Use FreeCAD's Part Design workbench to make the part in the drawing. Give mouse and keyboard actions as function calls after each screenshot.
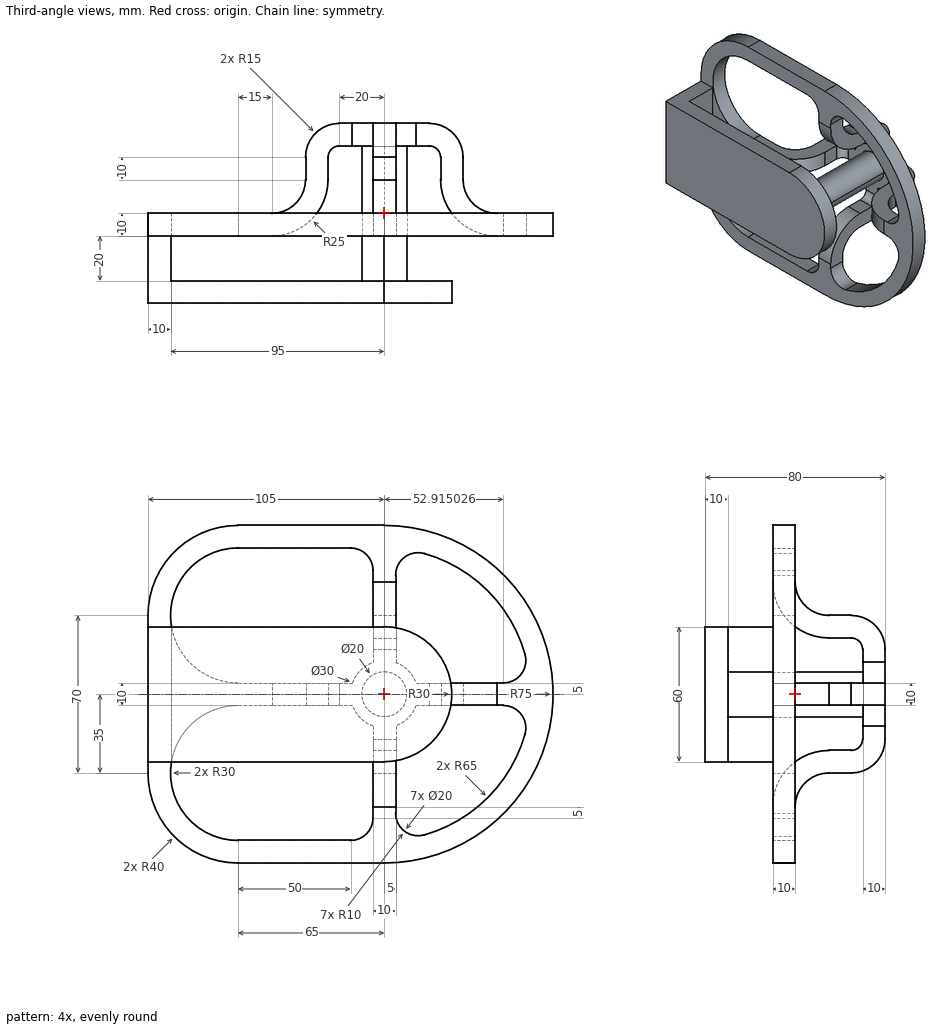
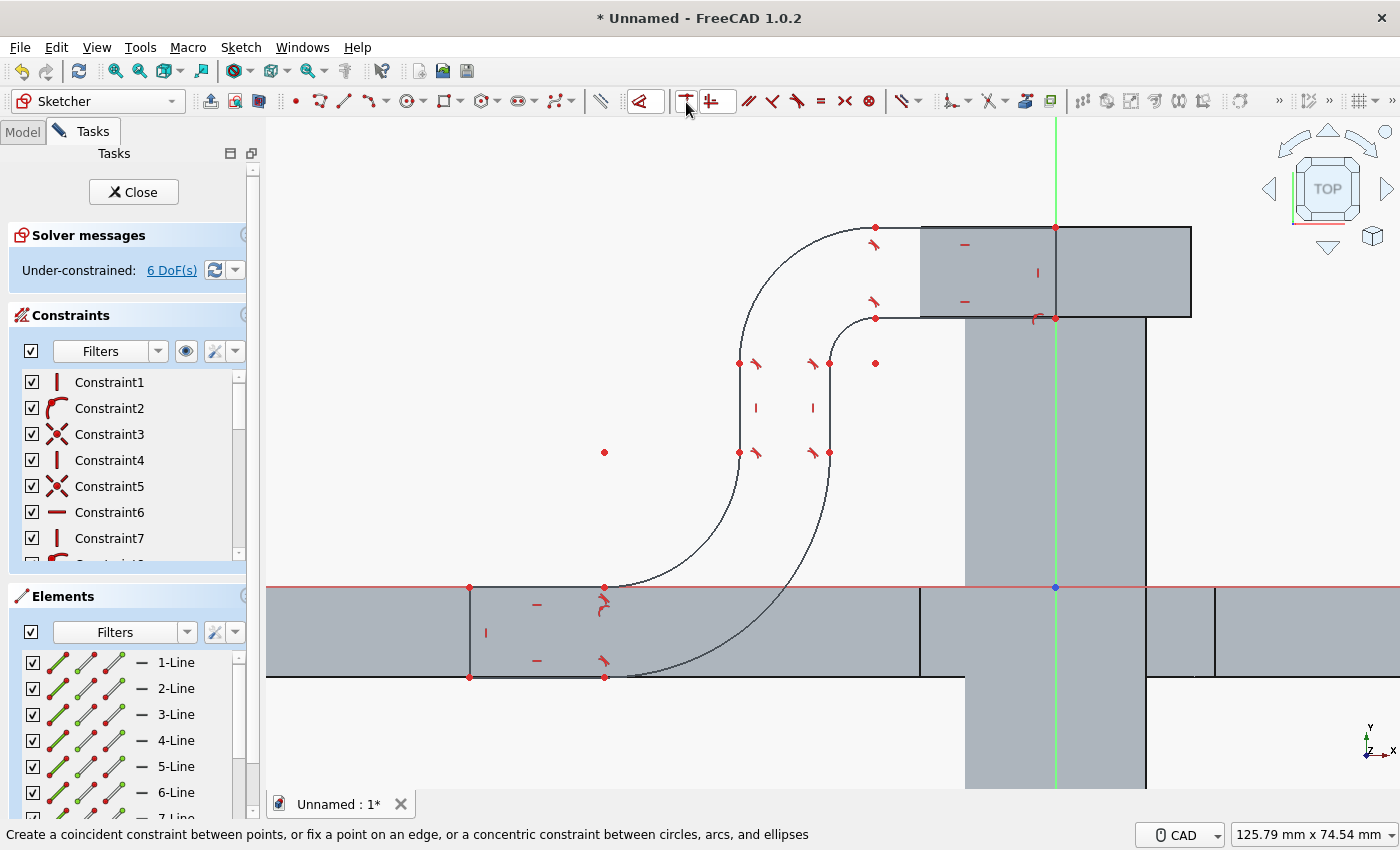
click(666, 573)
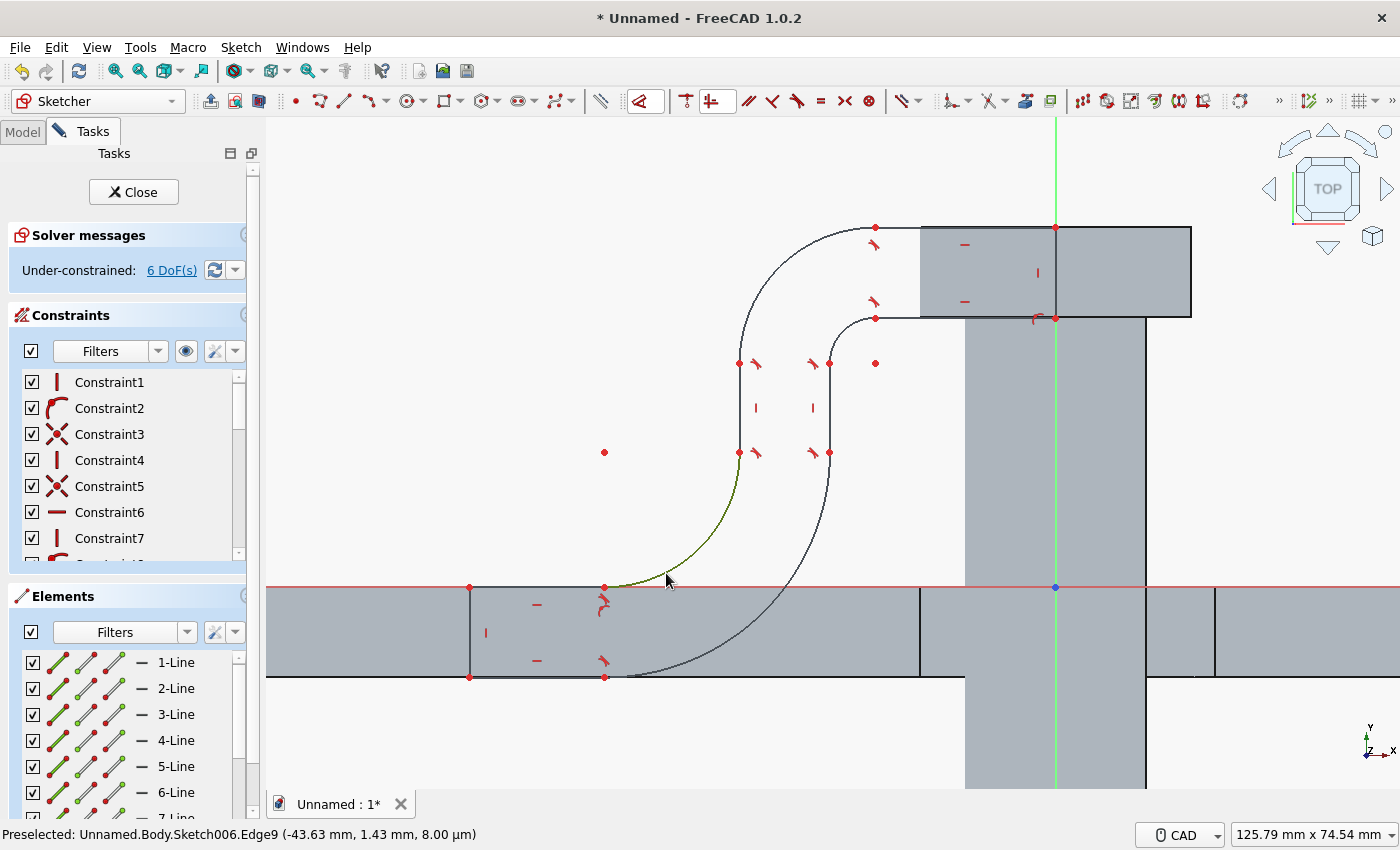
click(814, 242)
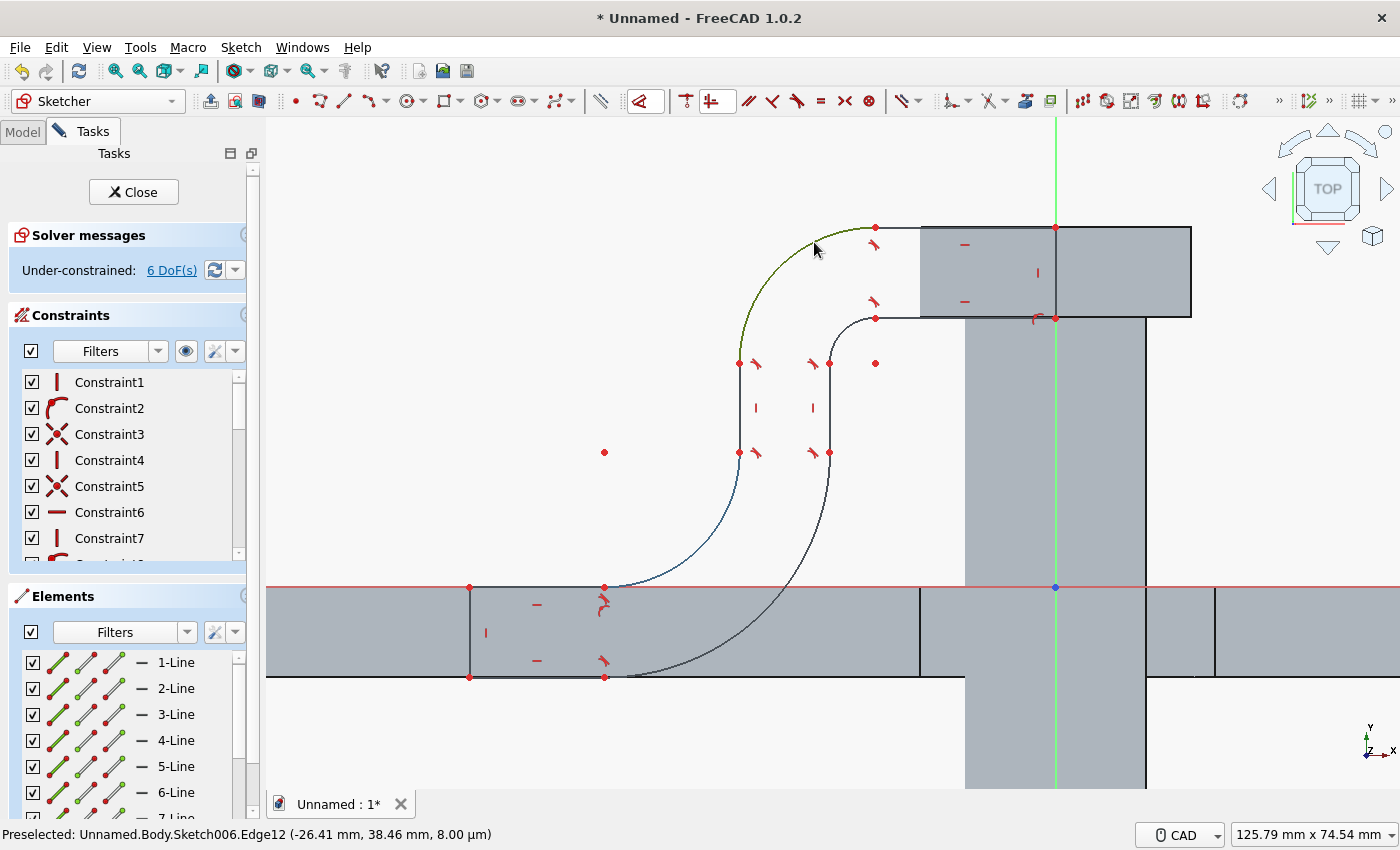
click(822, 102)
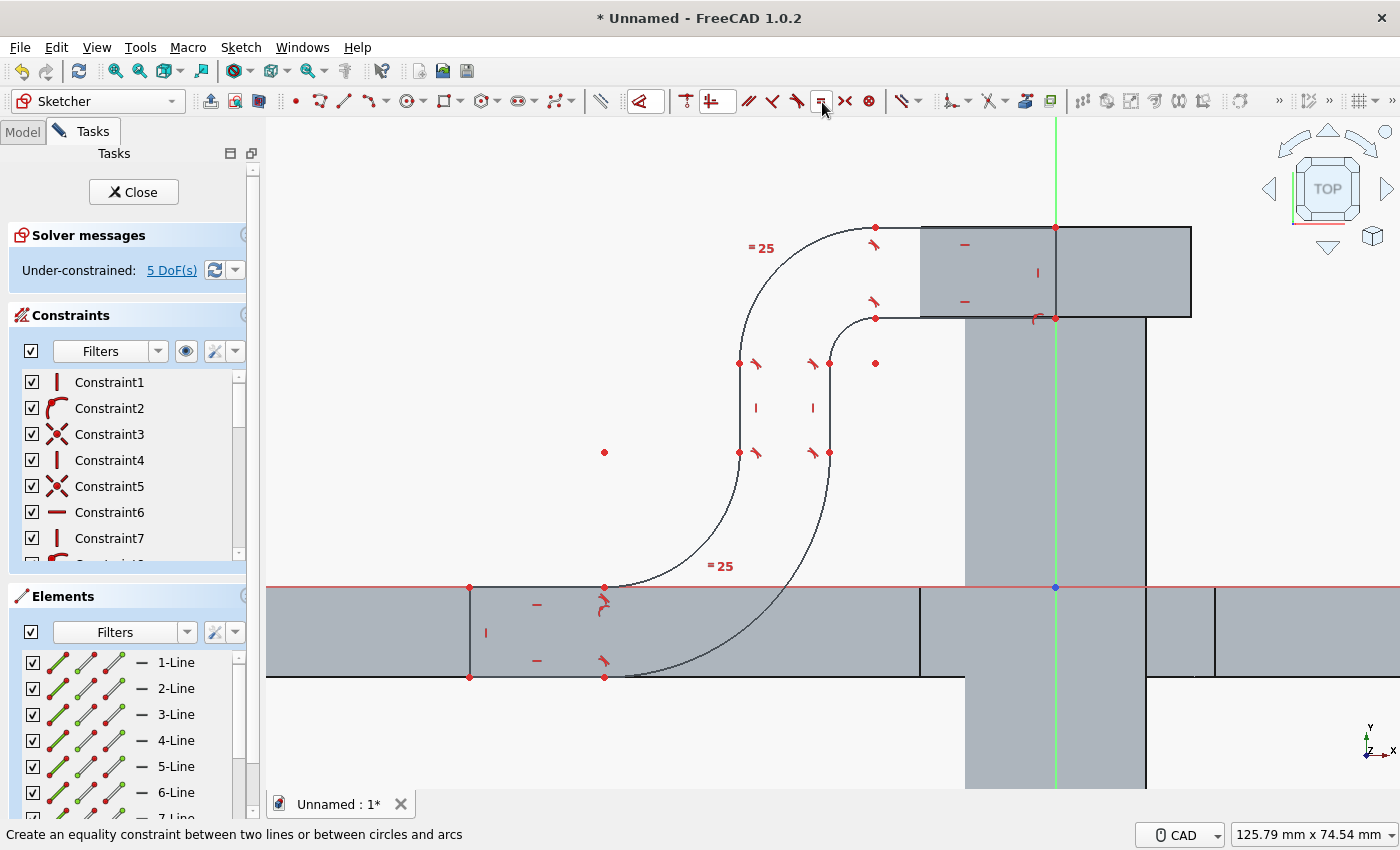
click(666, 573)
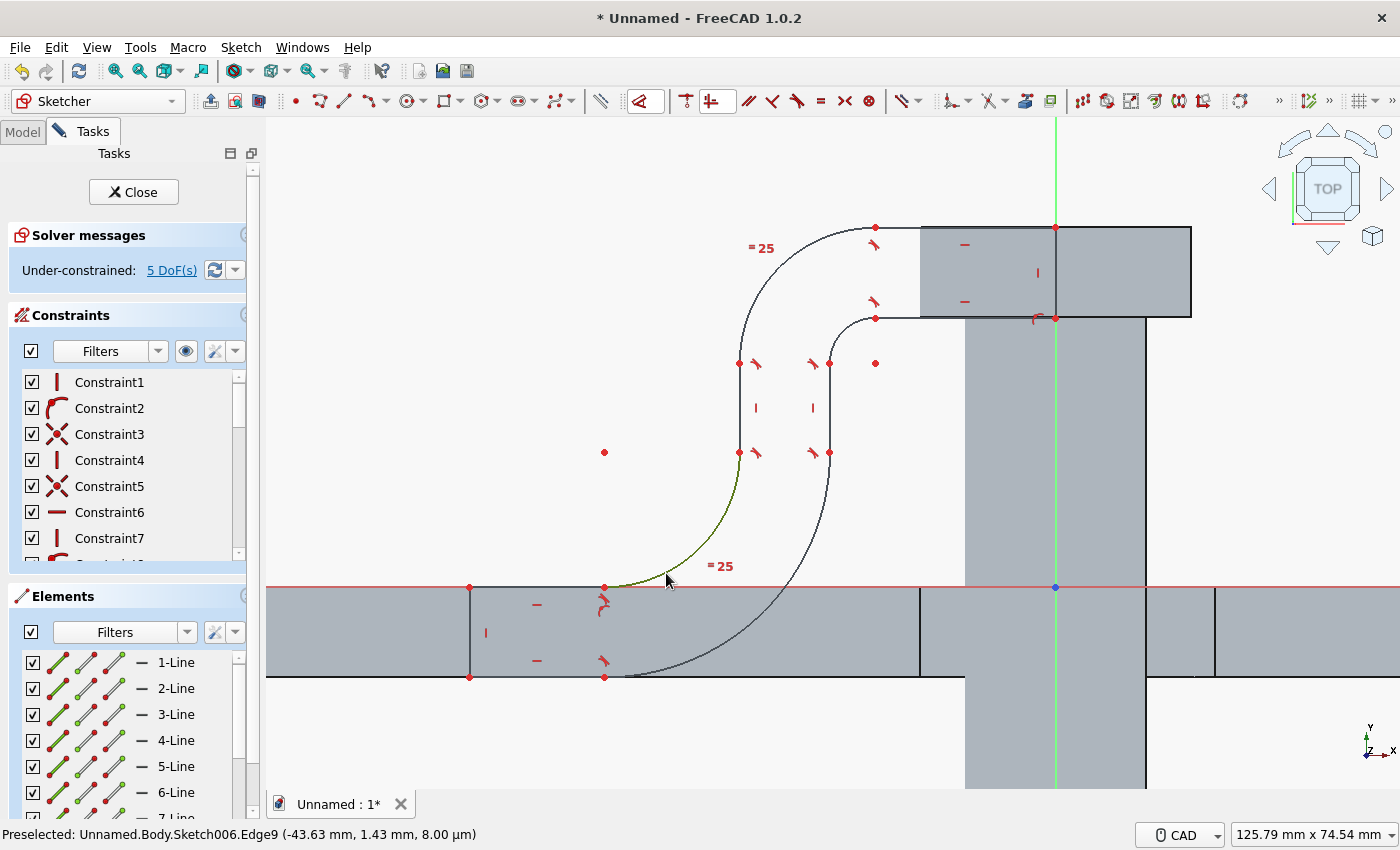
click(658, 102)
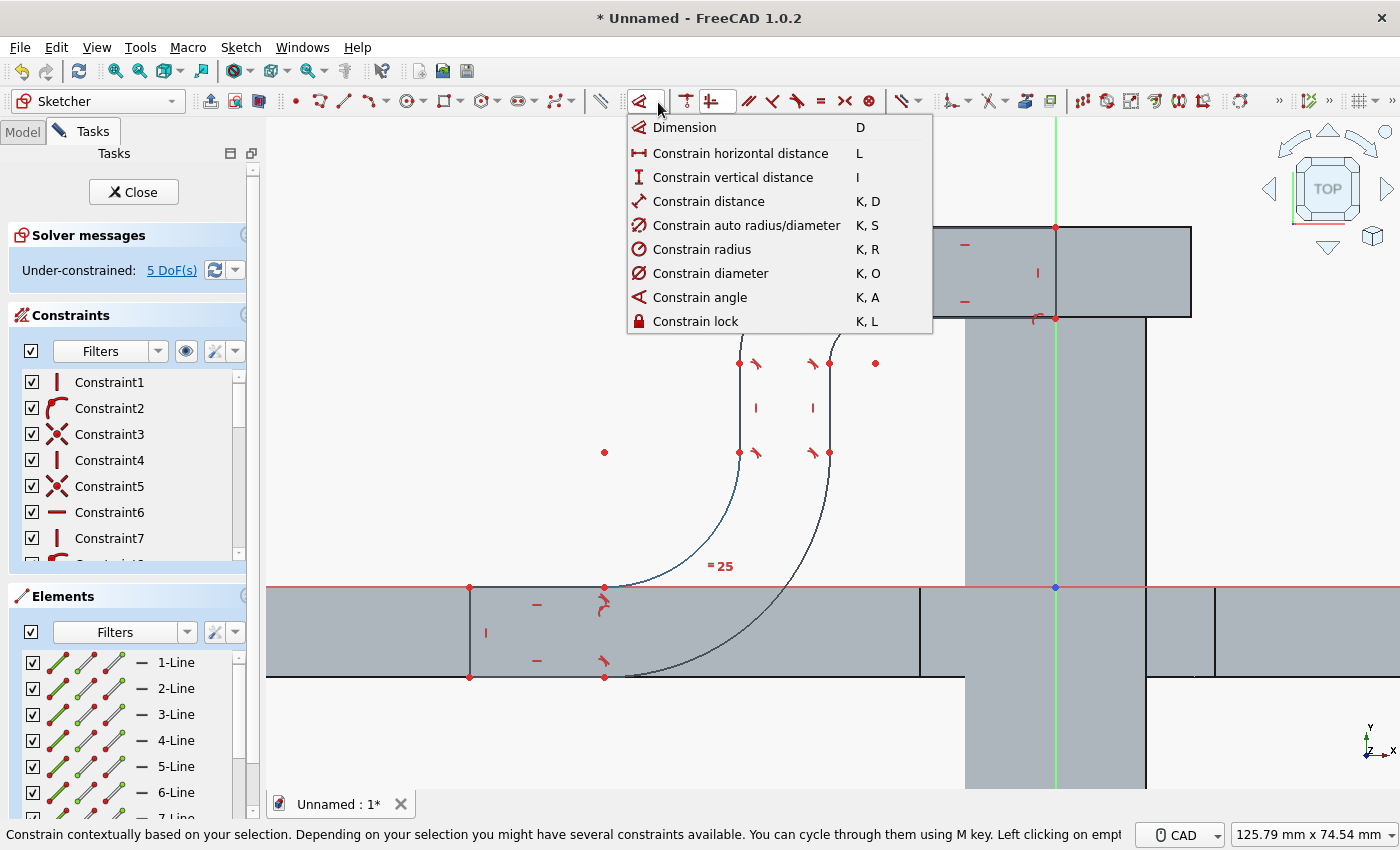
click(780, 249)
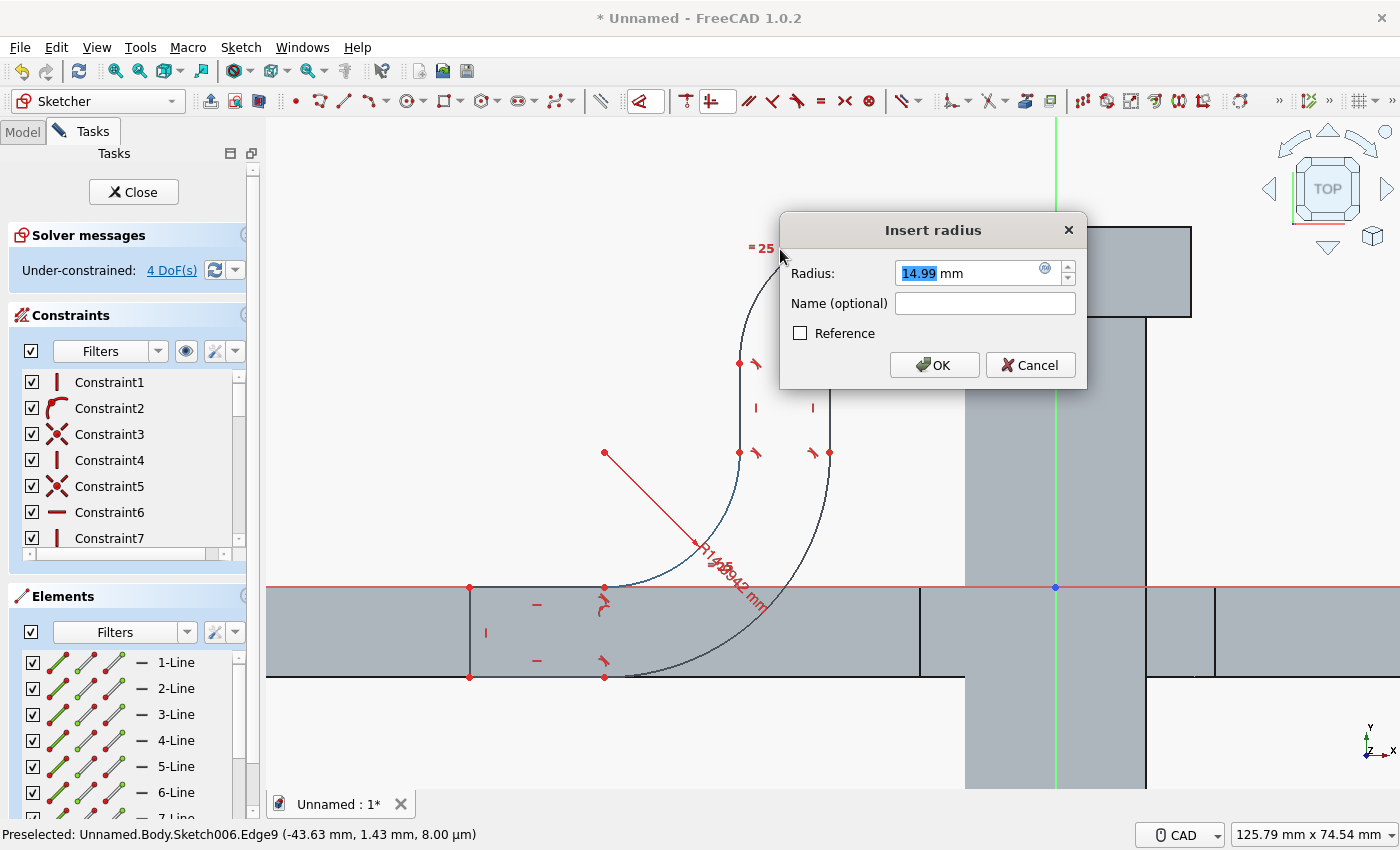
text(15)
key(Return)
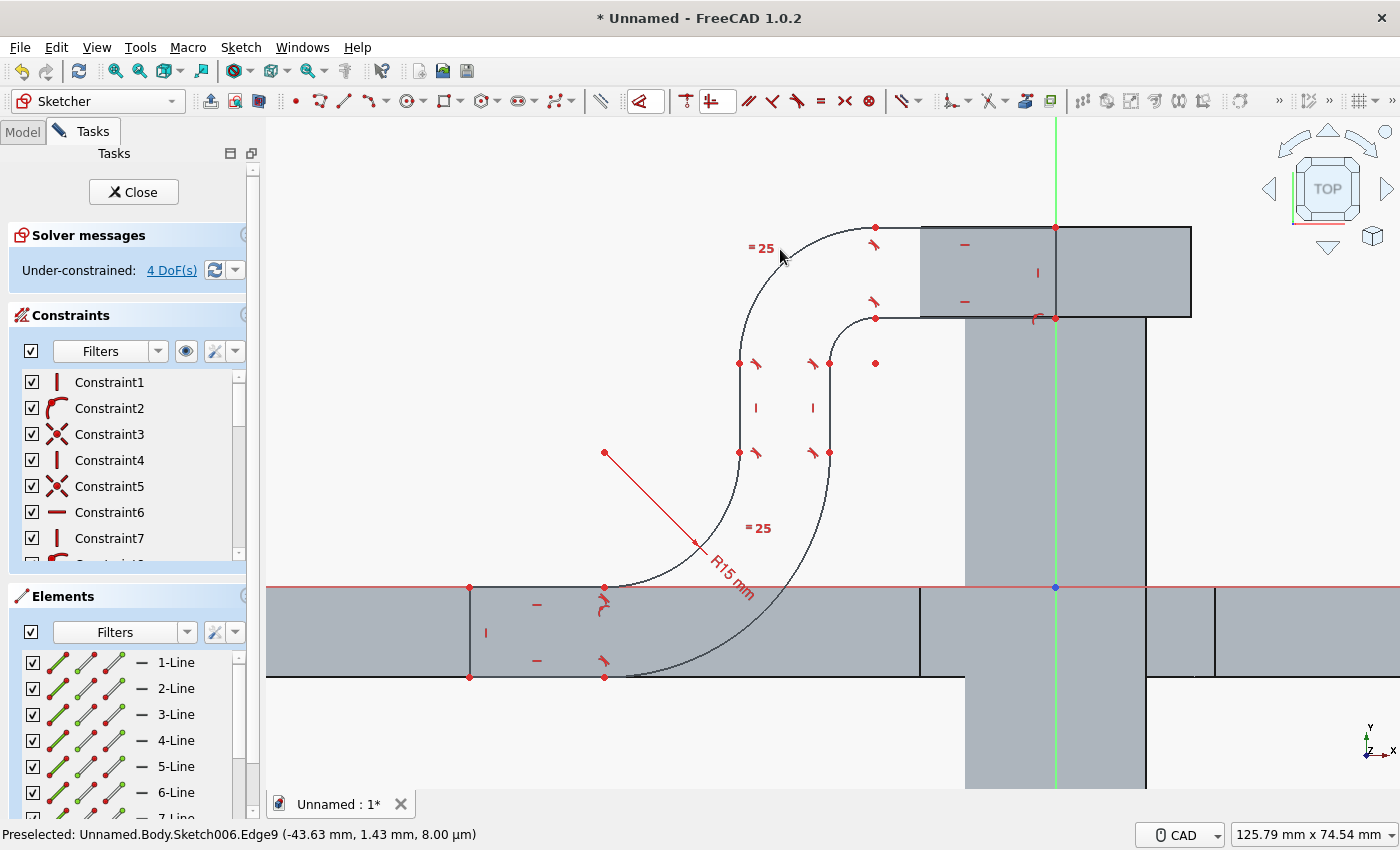
click(707, 653)